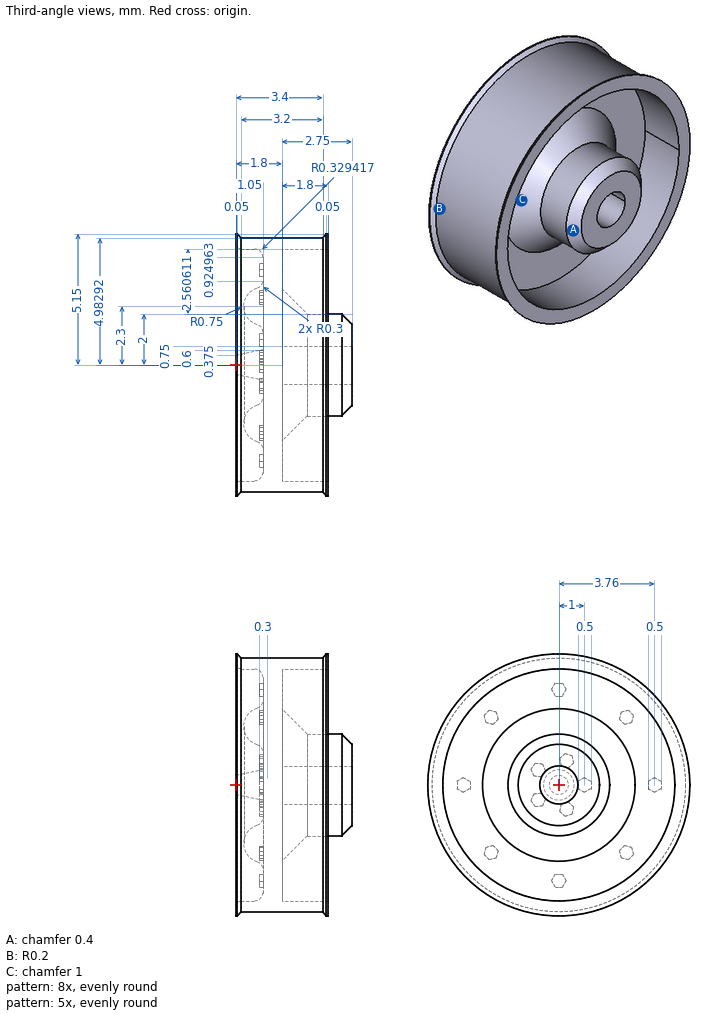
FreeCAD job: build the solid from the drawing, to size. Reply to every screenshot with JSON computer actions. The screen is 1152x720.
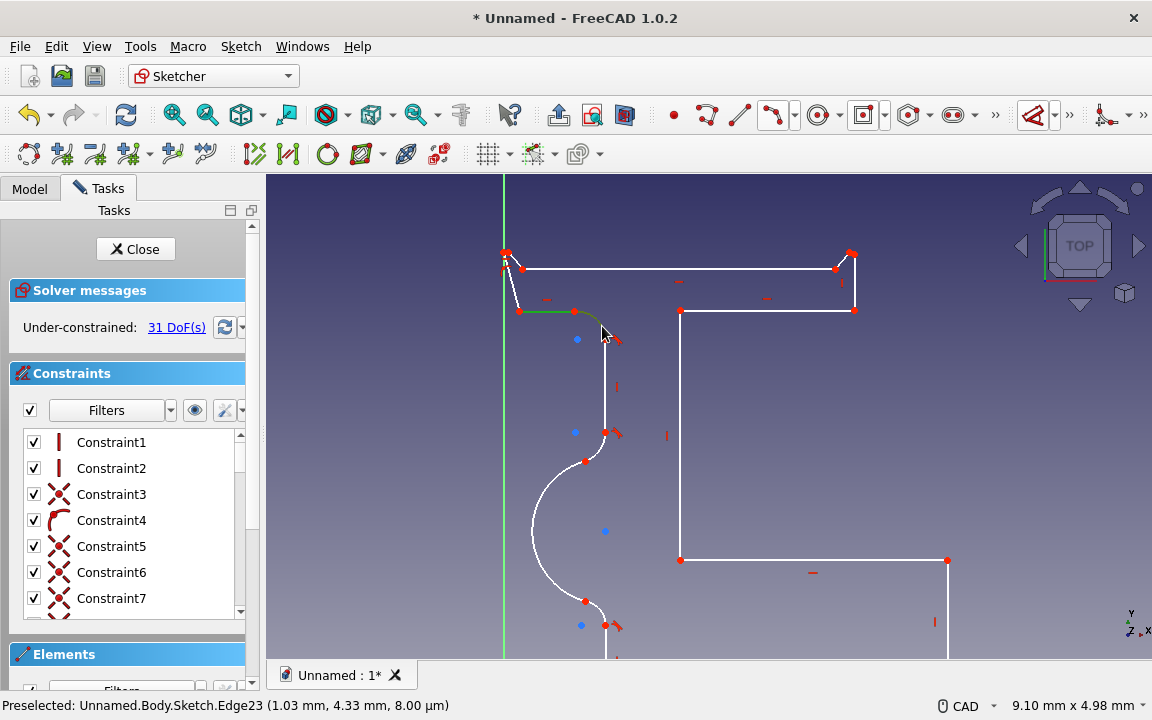
{"action": "key", "text": "t"}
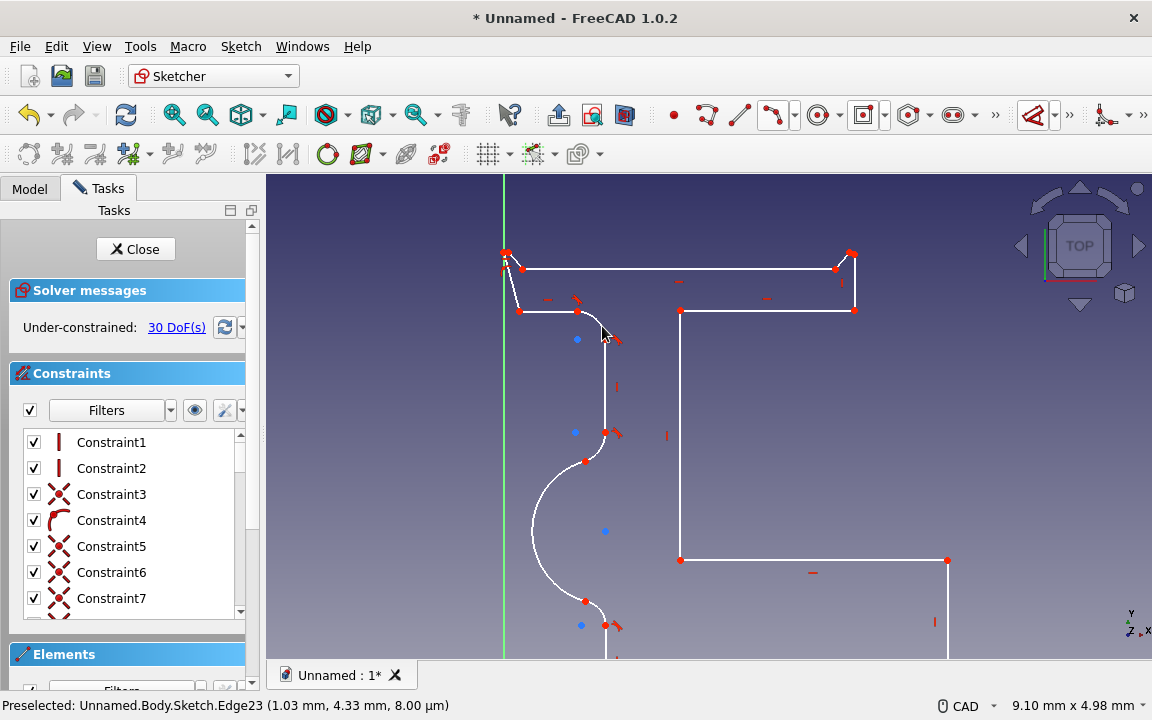
{"action": "scroll", "coordinate": [595, 456], "scroll_direction": "up", "scroll_amount": 2}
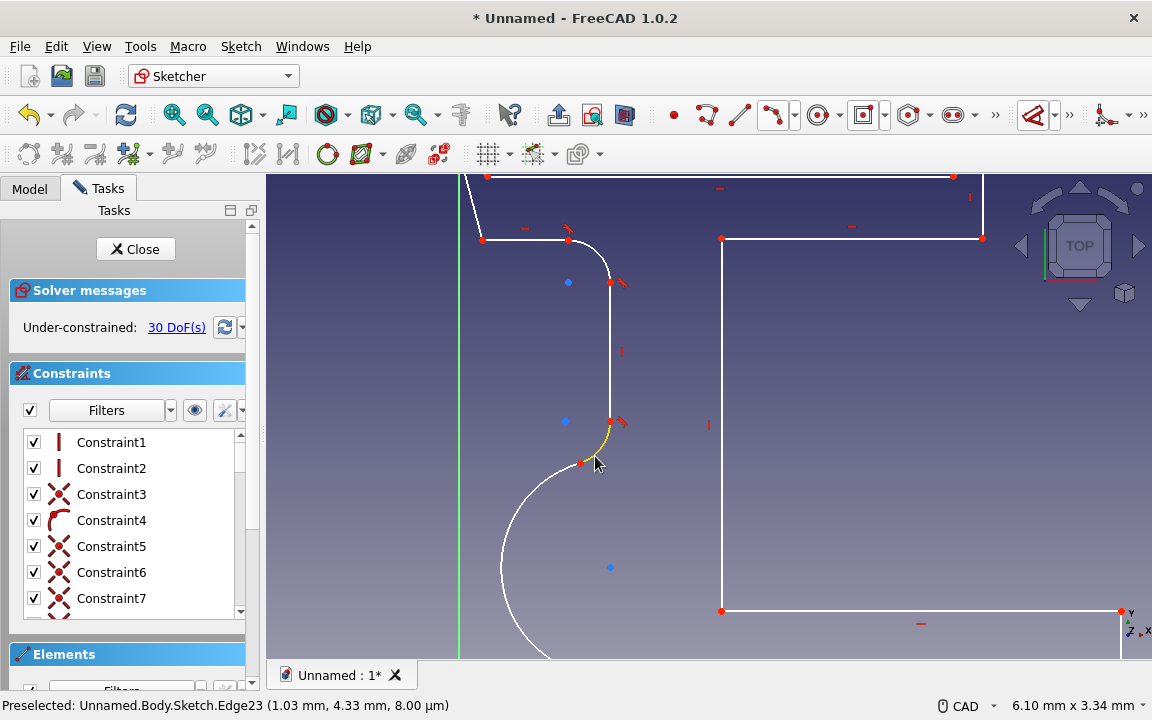
{"action": "left_click", "coordinate": [594, 455]}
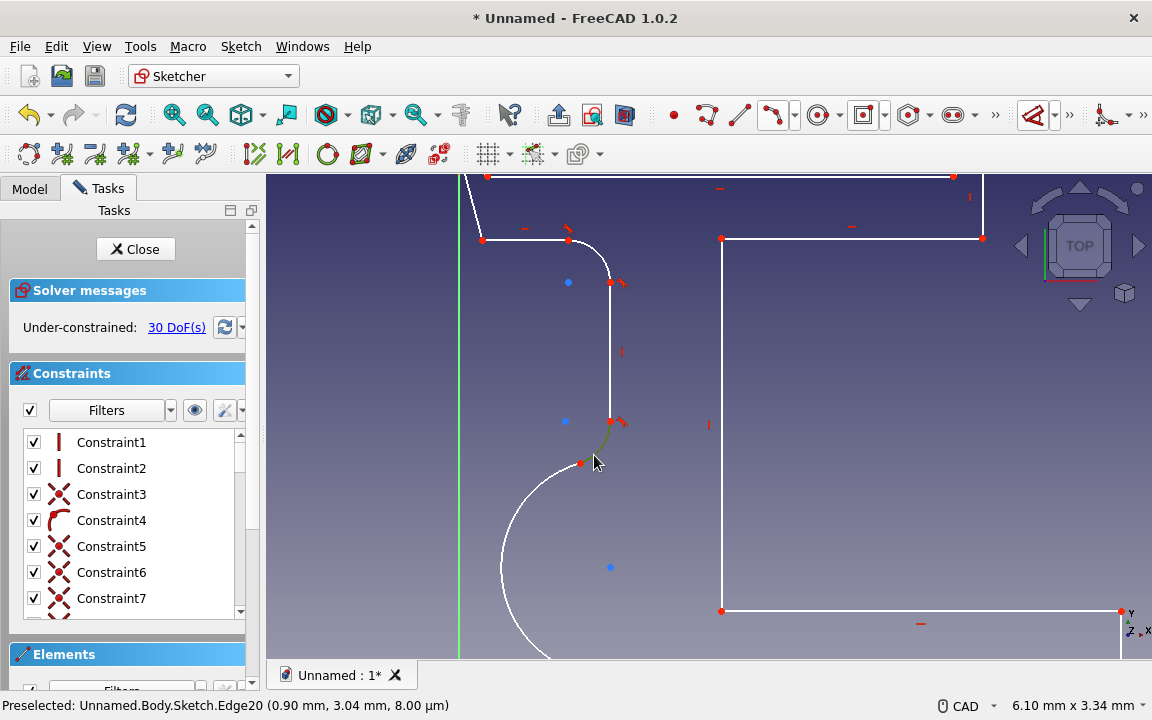
{"action": "left_click", "coordinate": [516, 514]}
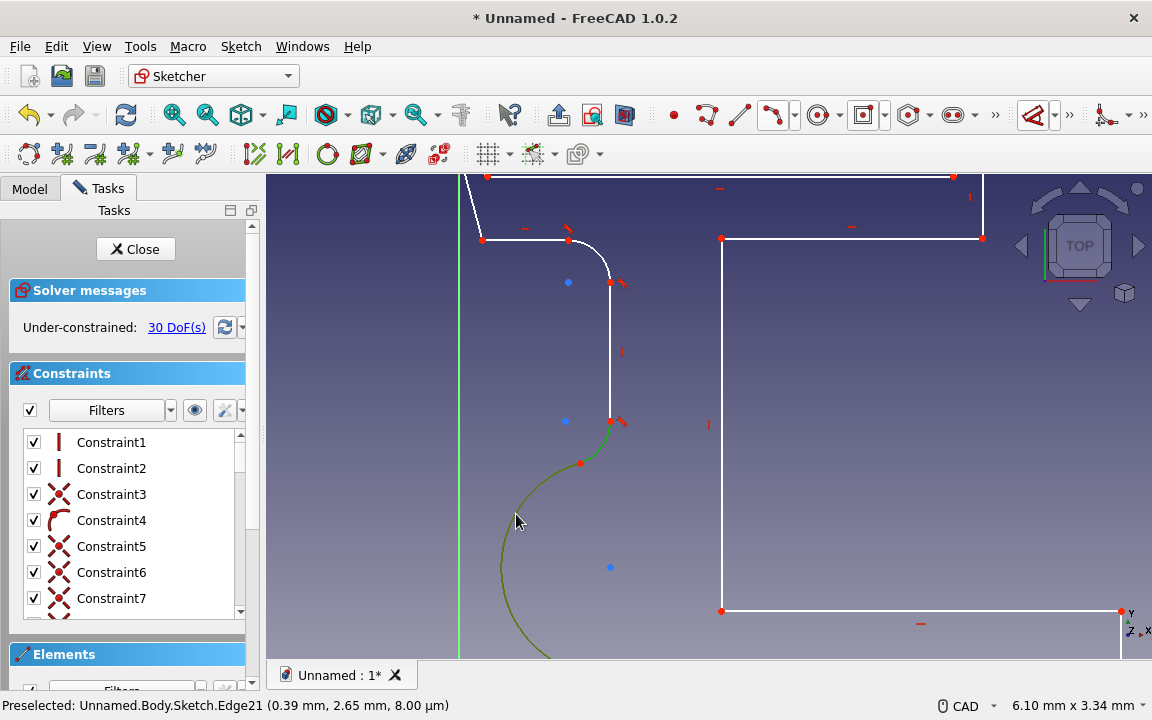
{"action": "key", "text": "t"}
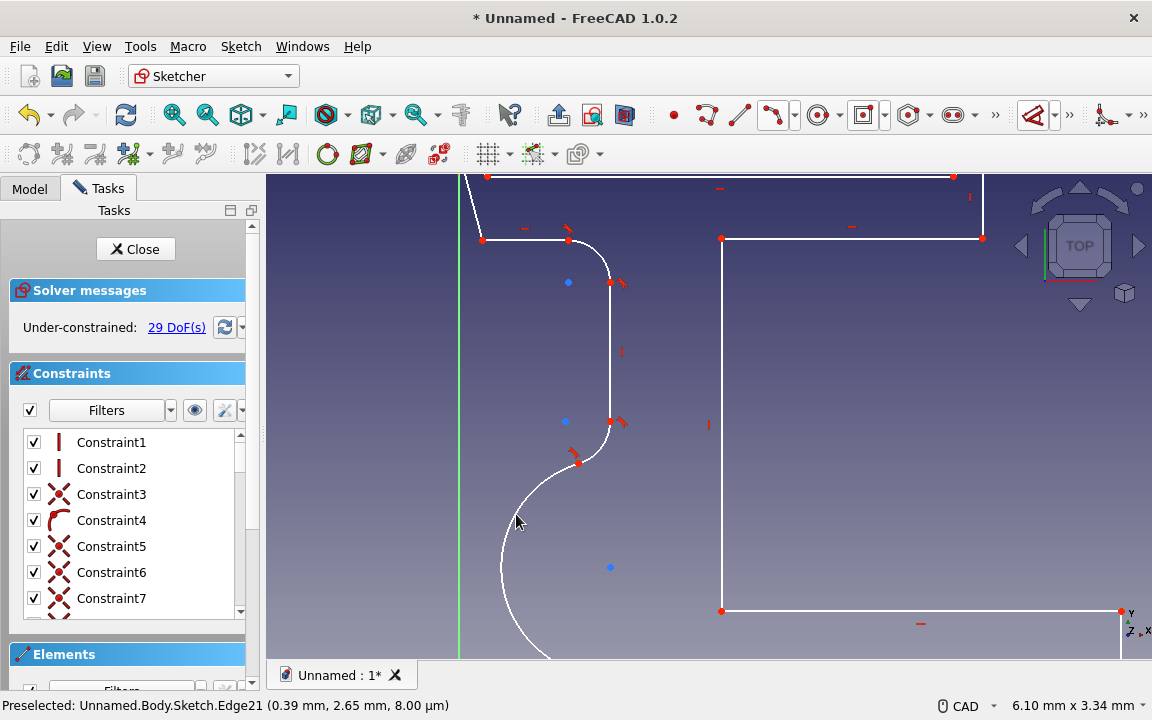
{"action": "left_click", "coordinate": [515, 515]}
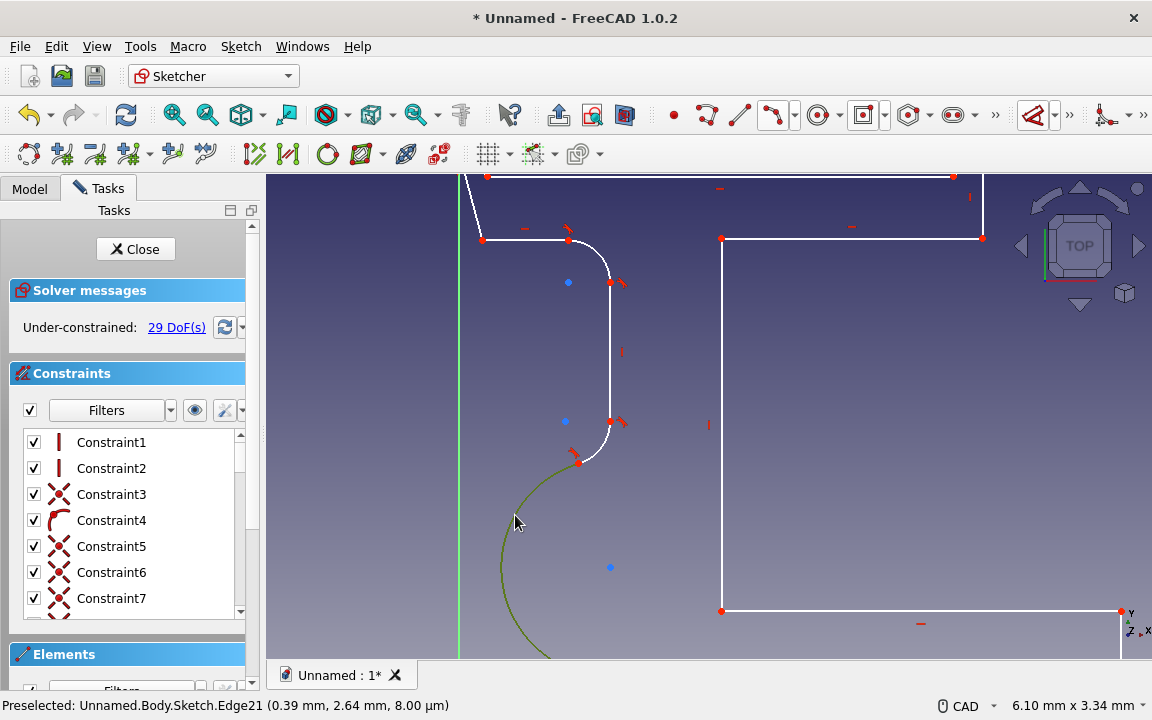
{"action": "scroll", "coordinate": [554, 353], "scroll_direction": "down", "scroll_amount": 5}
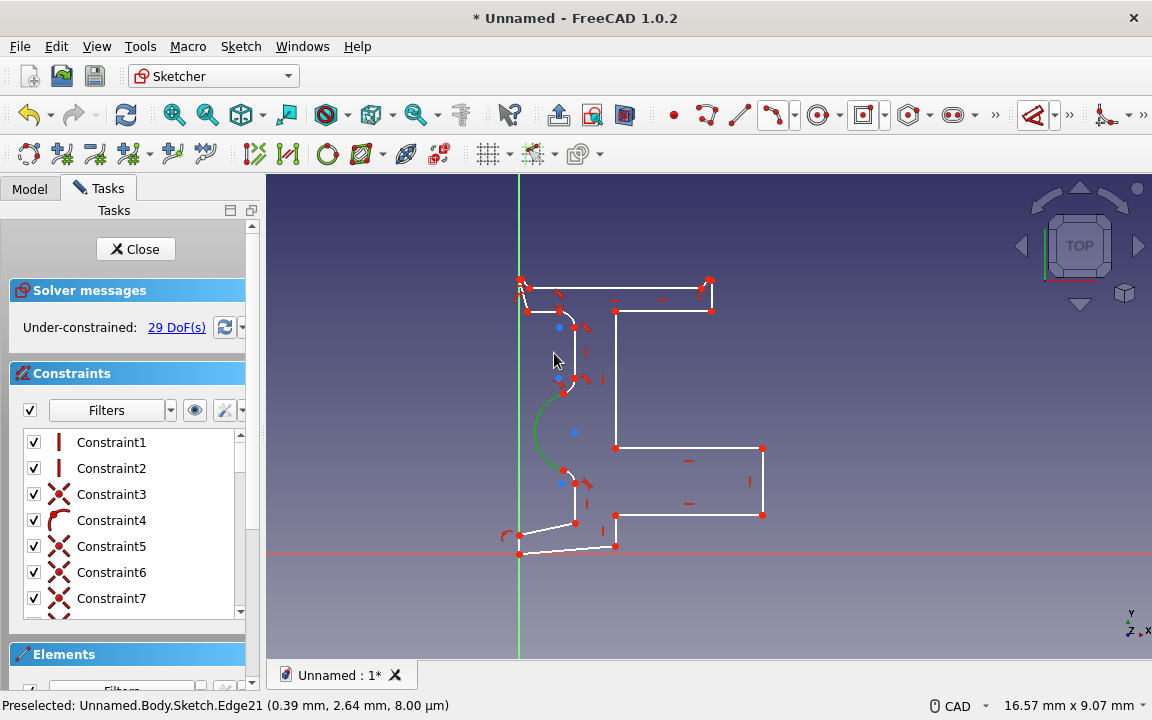
{"action": "scroll", "coordinate": [574, 478], "scroll_direction": "up", "scroll_amount": 5}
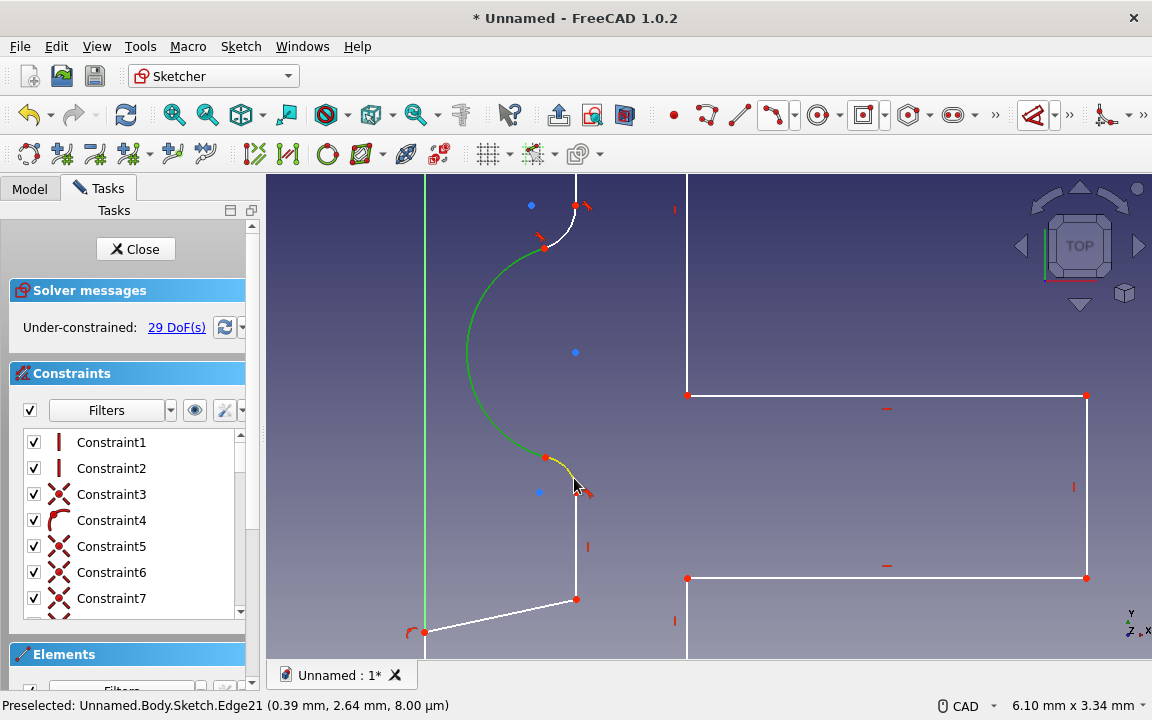
{"action": "left_click", "coordinate": [573, 478]}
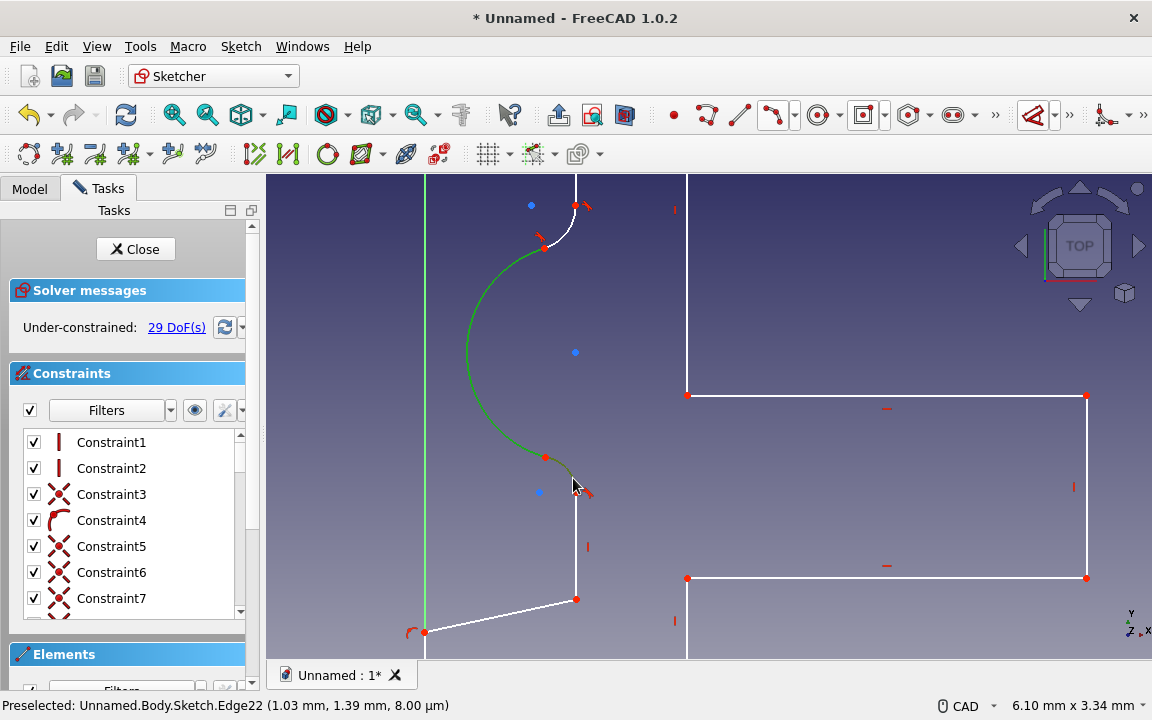
{"action": "key", "text": "t"}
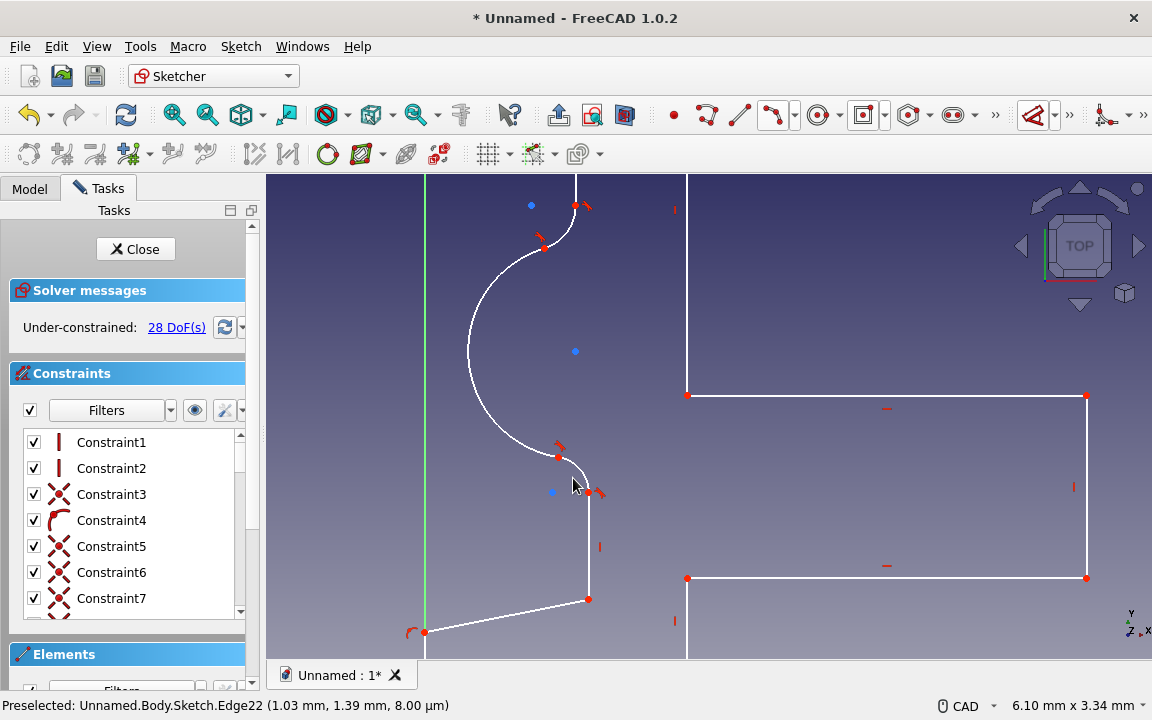
{"action": "scroll", "coordinate": [574, 478], "scroll_direction": "down", "scroll_amount": 5}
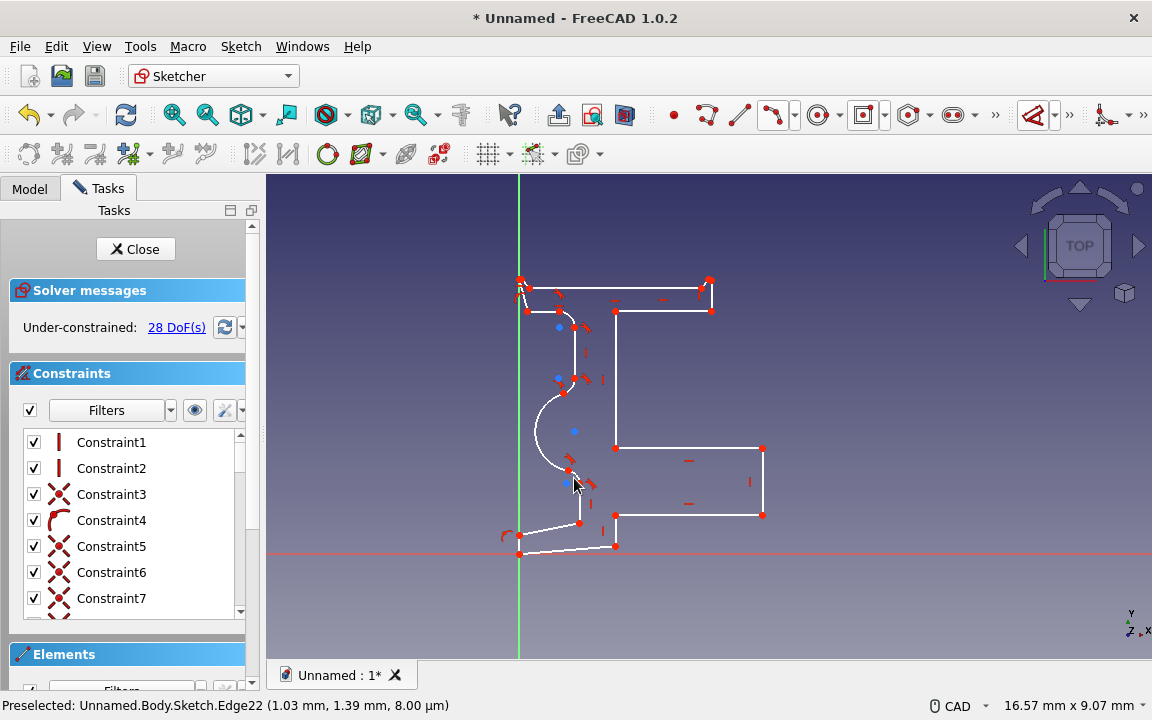
{"action": "scroll", "coordinate": [587, 549], "scroll_direction": "up", "scroll_amount": 5}